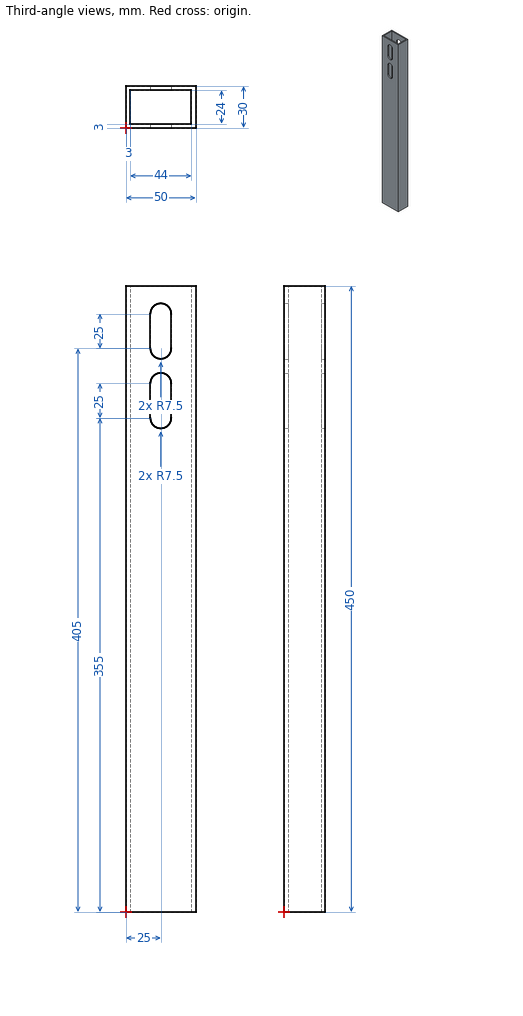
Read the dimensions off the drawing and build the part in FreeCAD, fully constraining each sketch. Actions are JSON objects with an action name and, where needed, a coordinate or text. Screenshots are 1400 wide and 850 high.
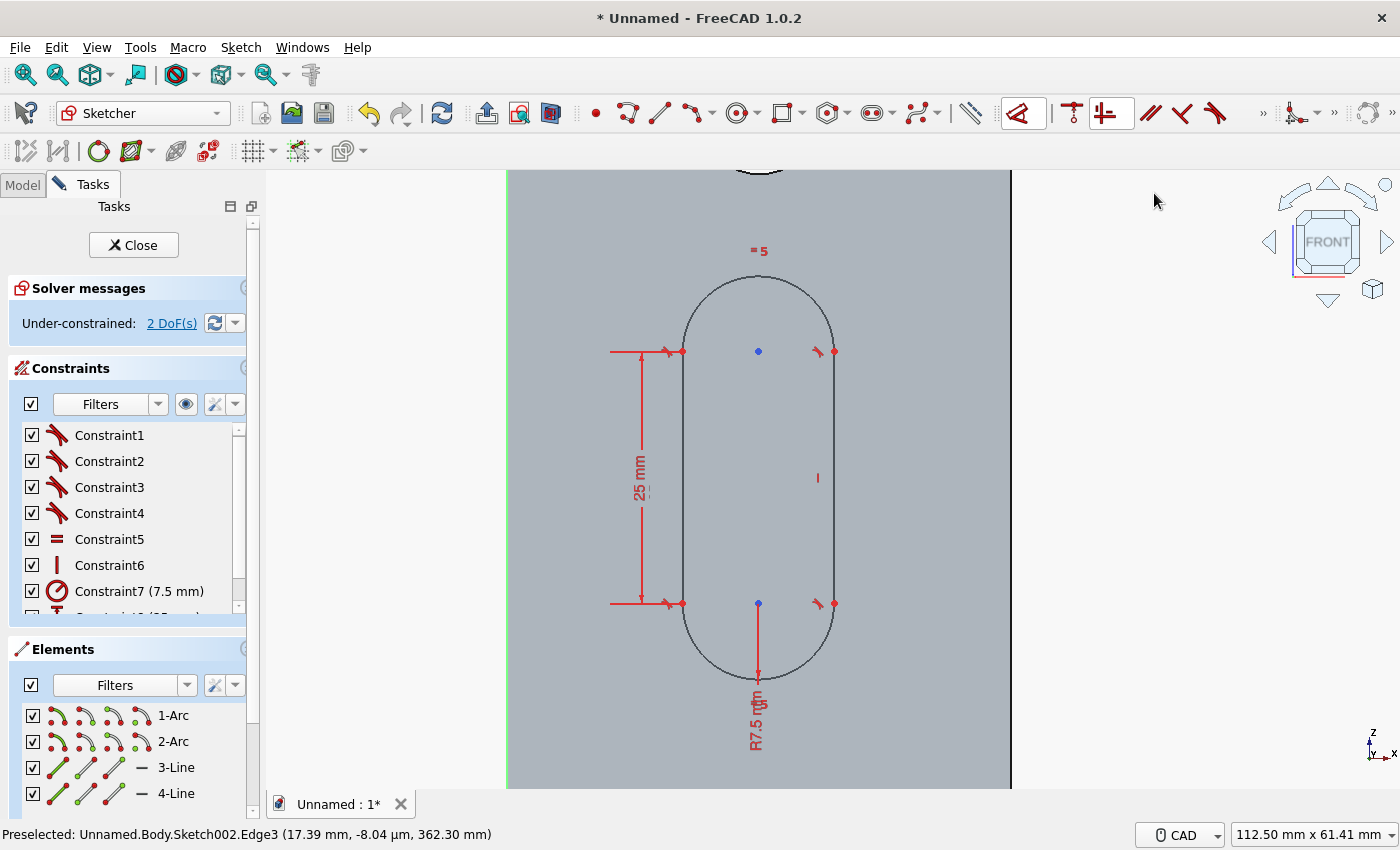
{"action": "left_click", "coordinate": [758, 604]}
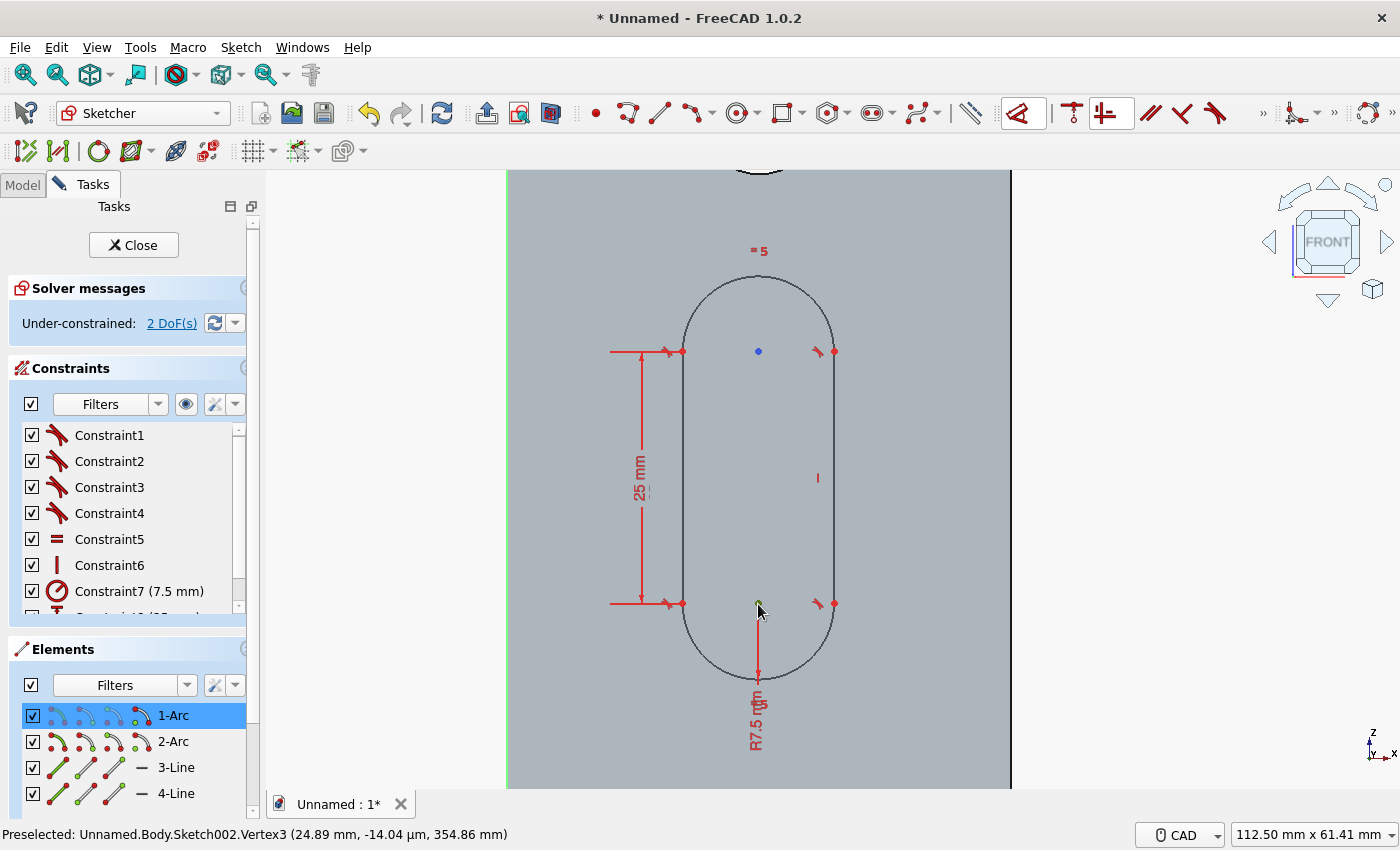
{"action": "left_click", "coordinate": [1040, 114]}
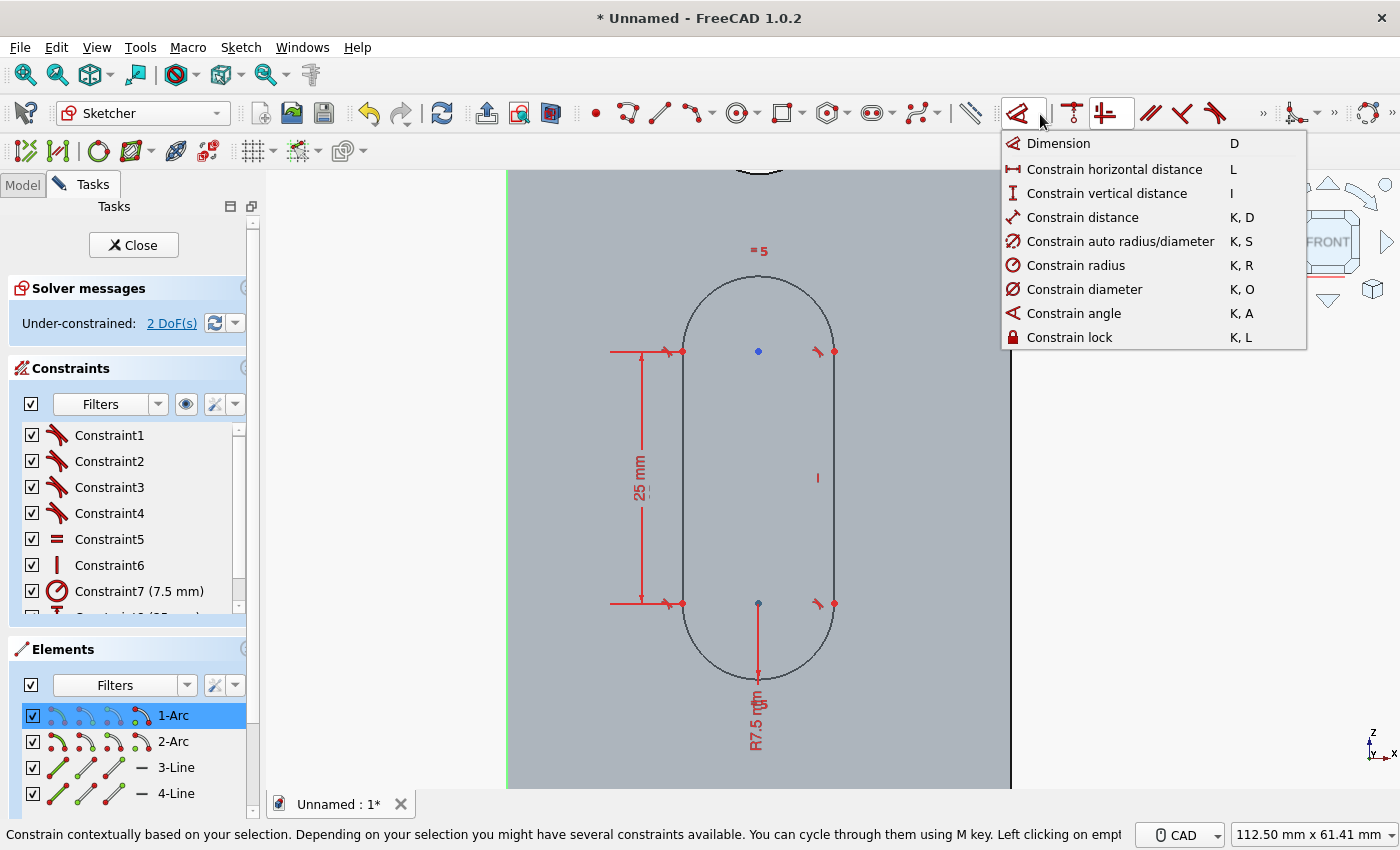
{"action": "left_click", "coordinate": [1154, 169]}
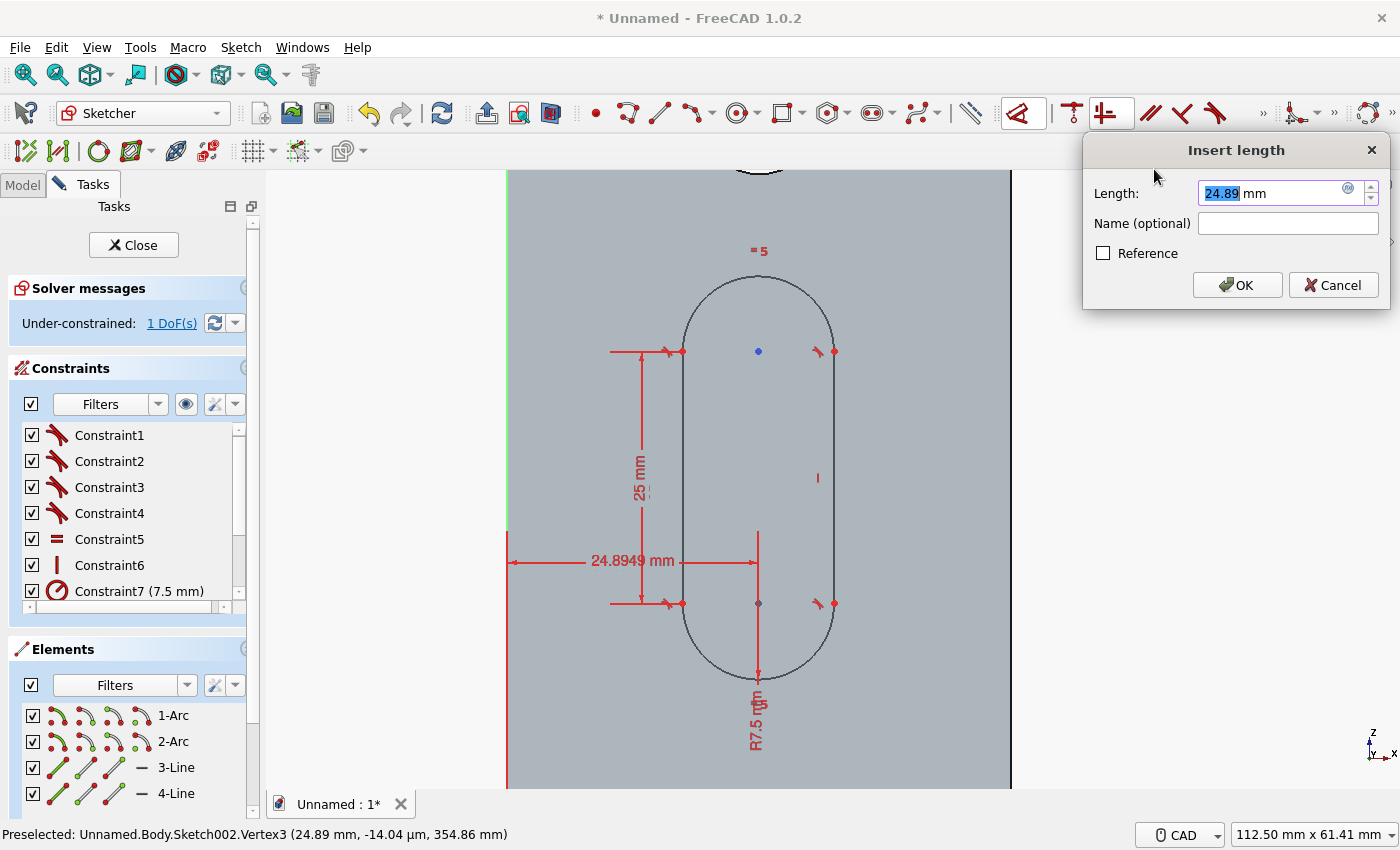
{"action": "type", "text": "25"}
{"action": "key", "text": "Return"}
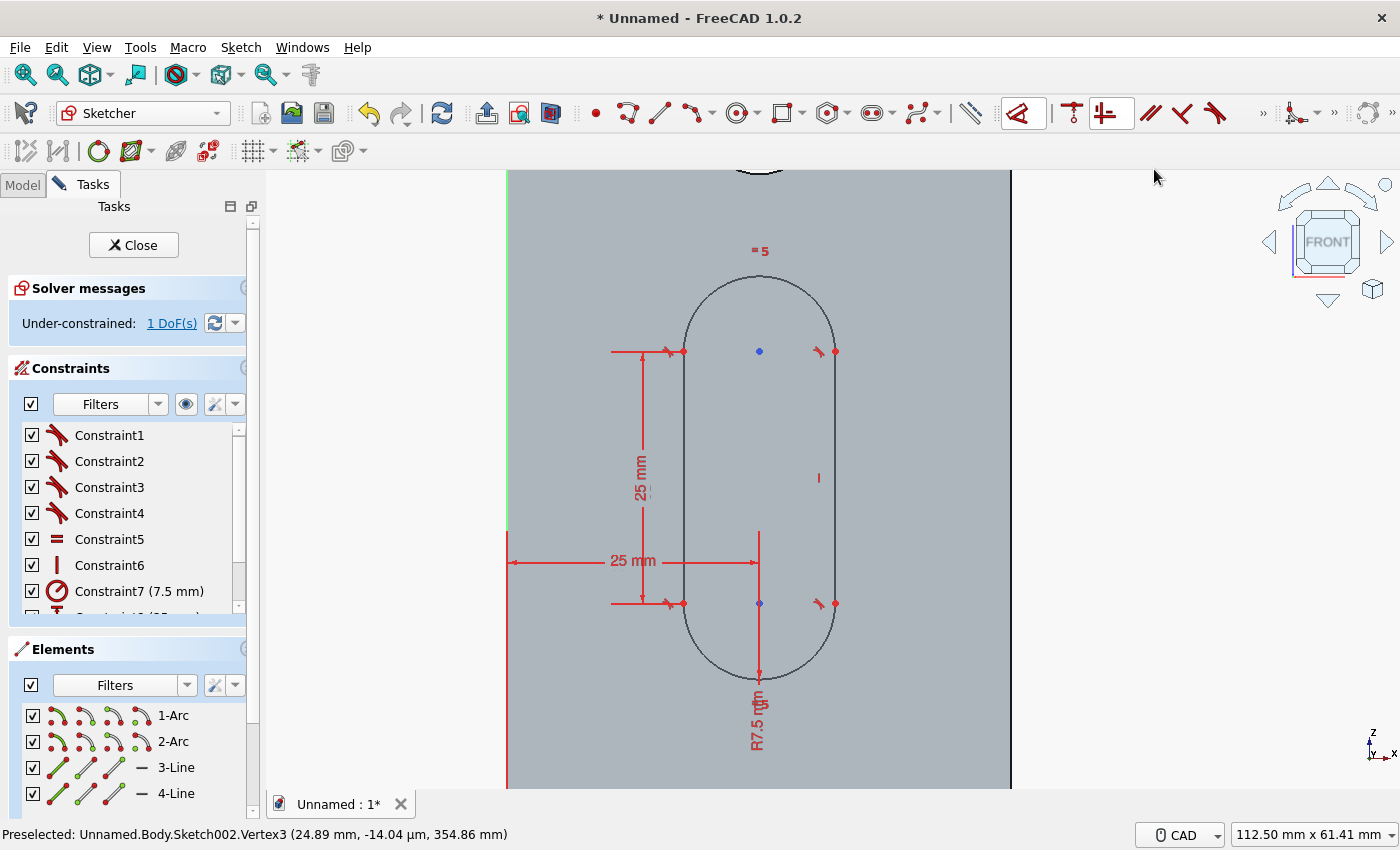
{"action": "left_click", "coordinate": [684, 604]}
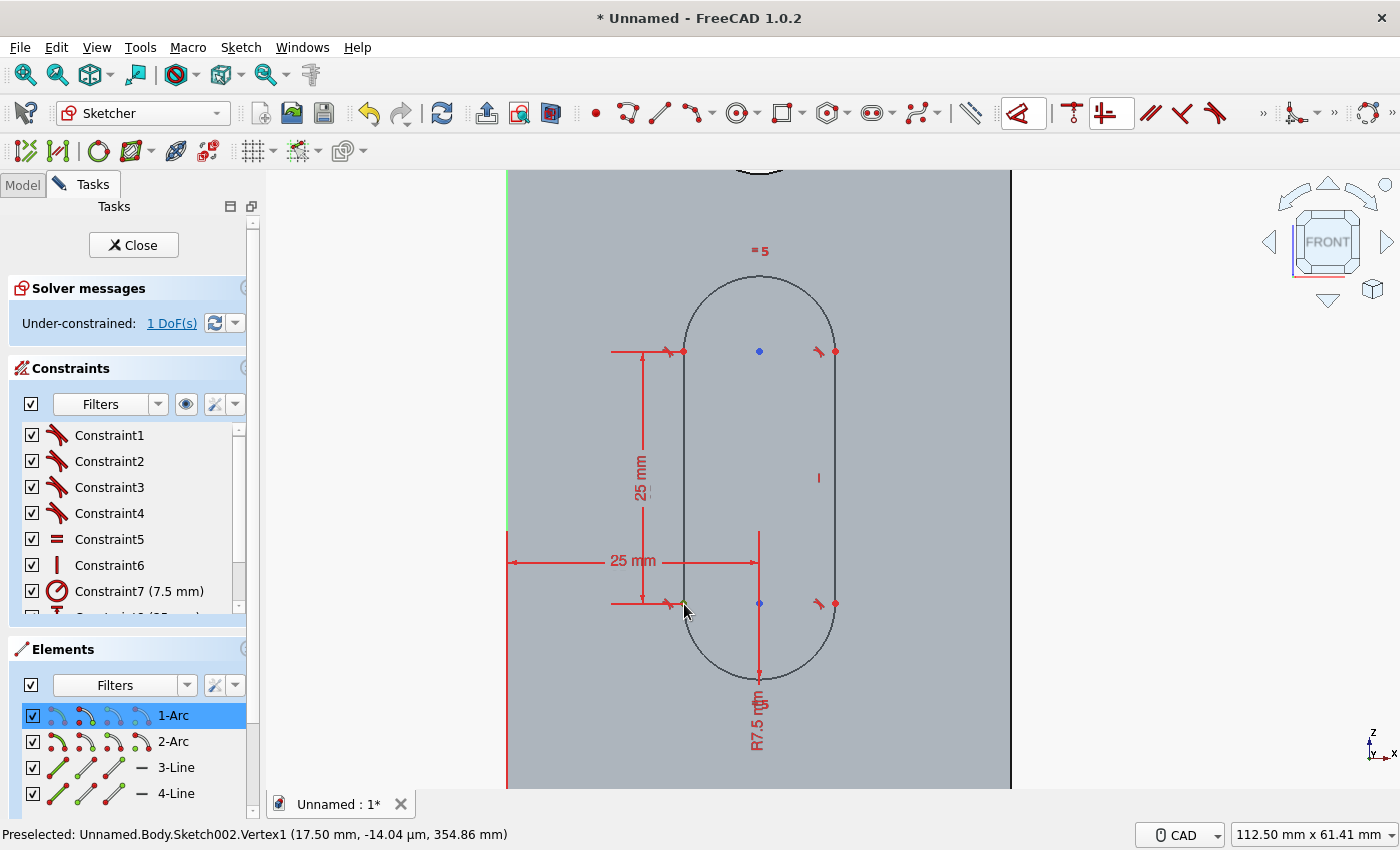
{"action": "key", "text": "i"}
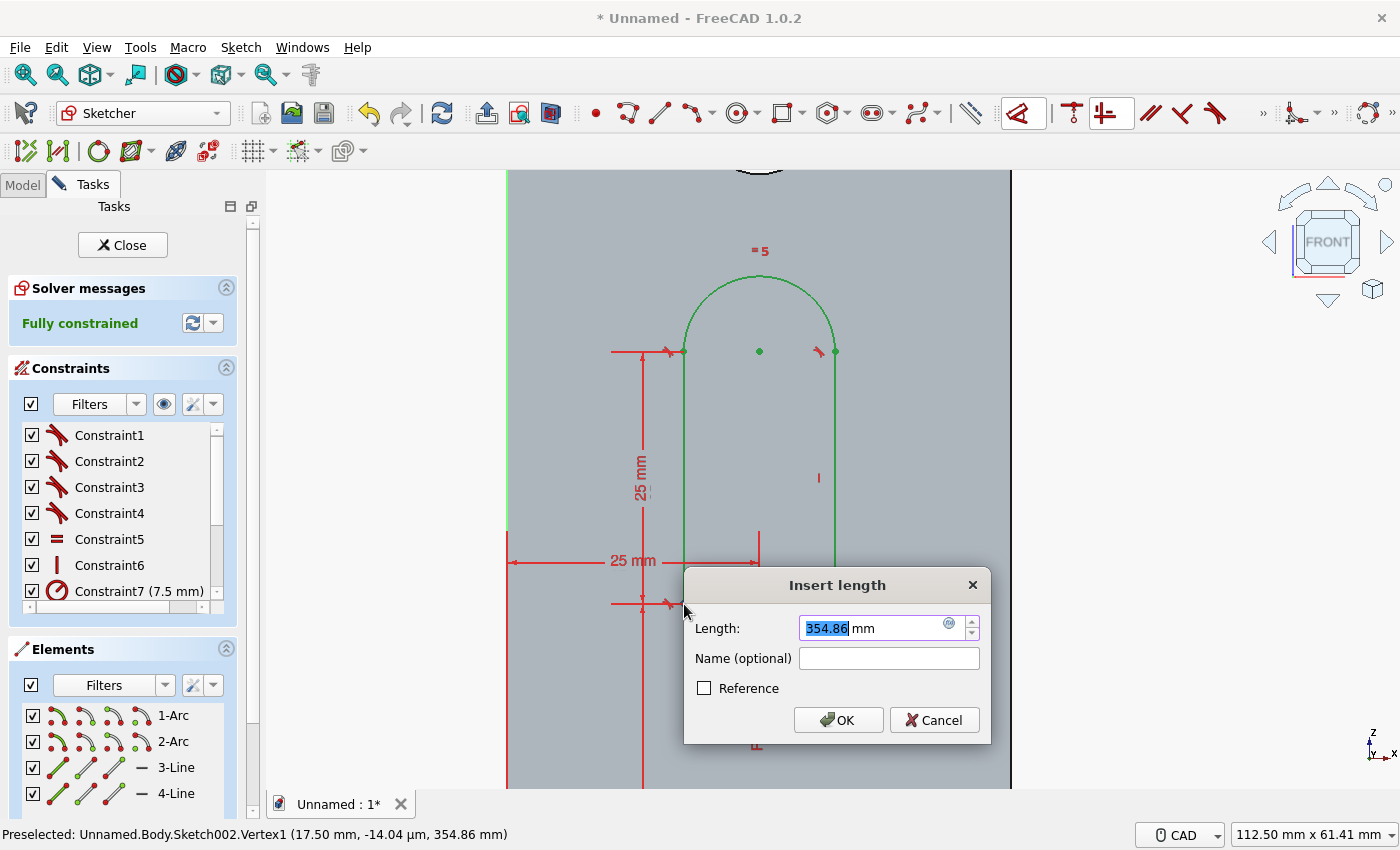
{"action": "type", "text": "355"}
{"action": "key", "text": "Return"}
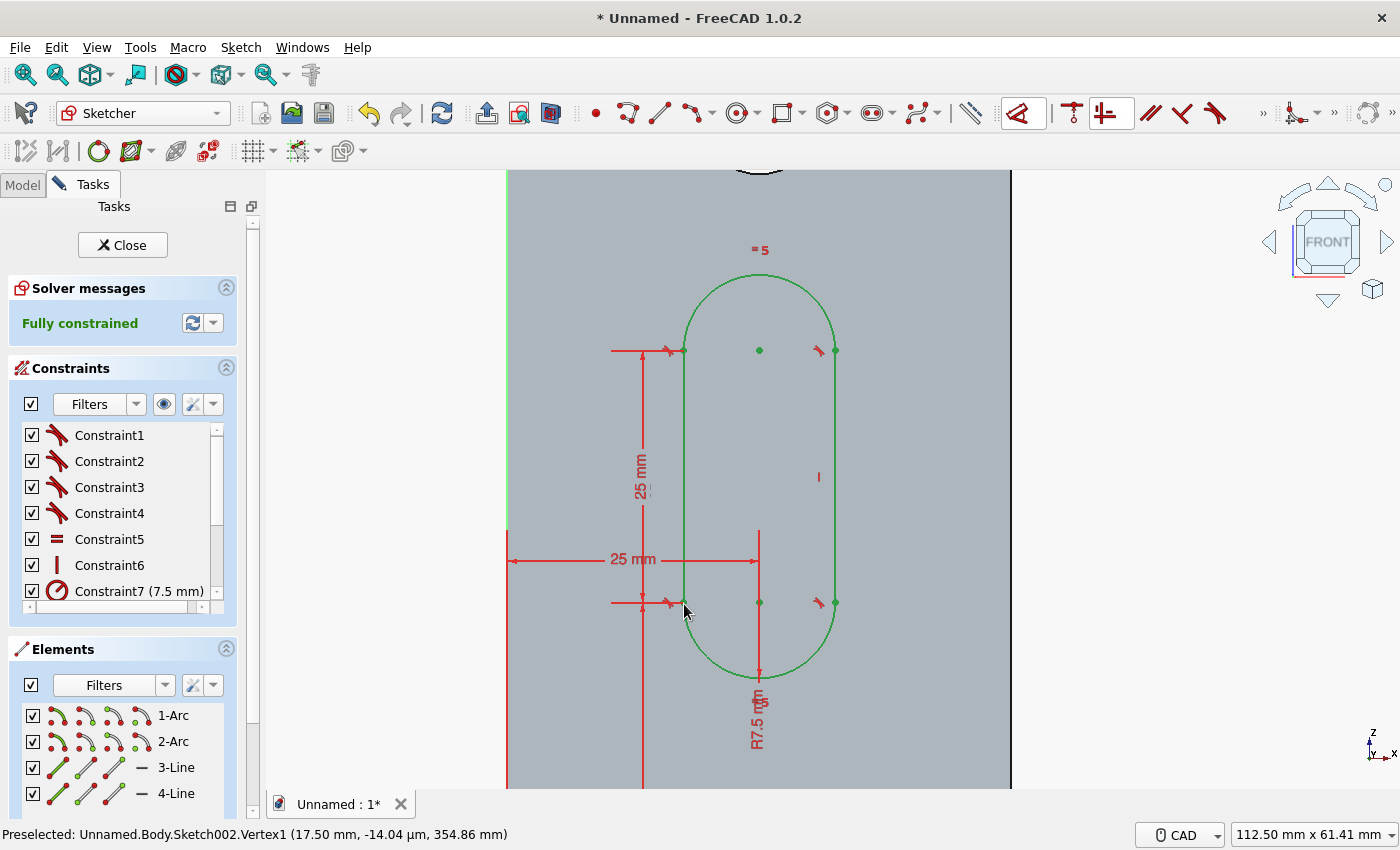
{"action": "left_click", "coordinate": [123, 245]}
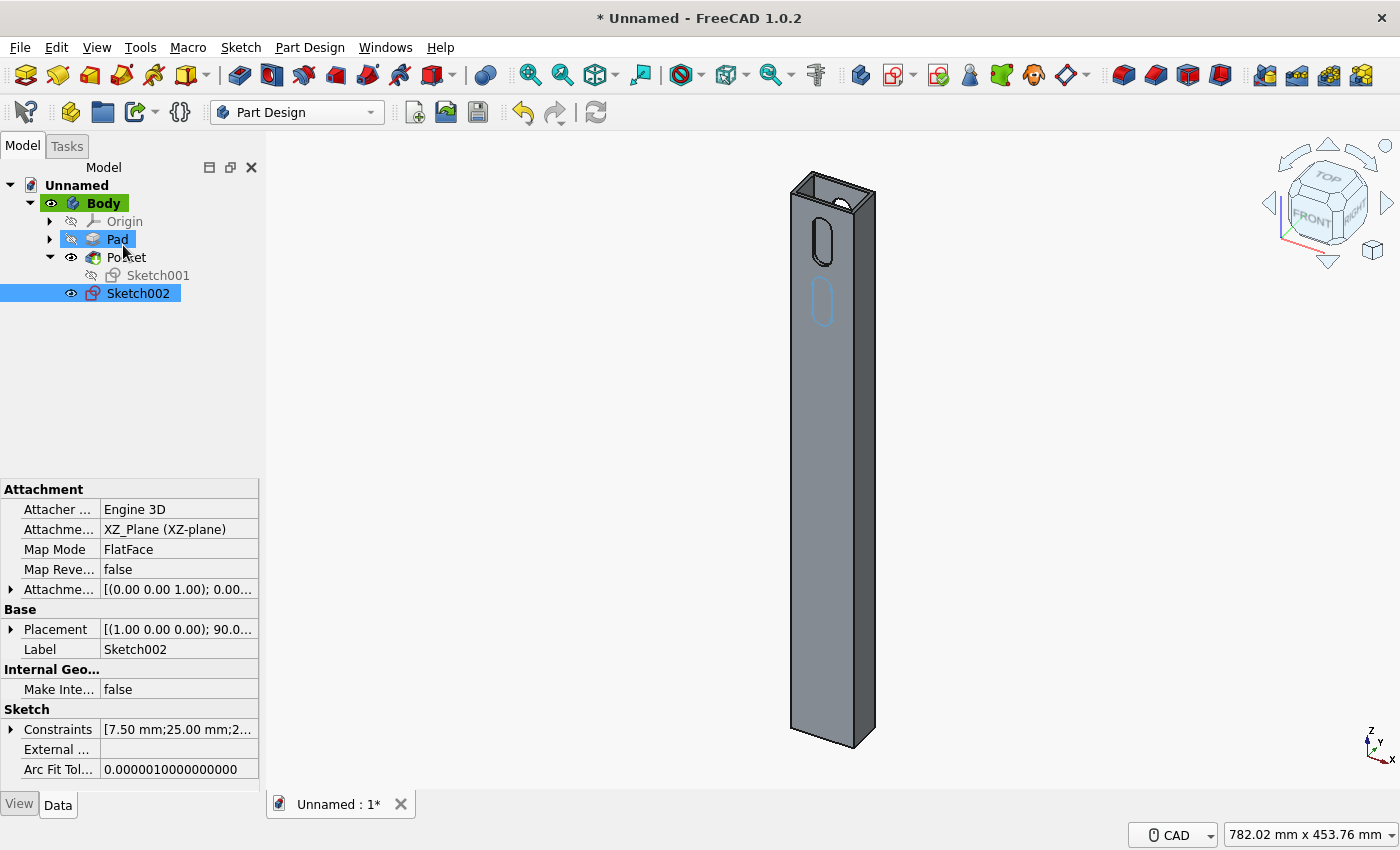
{"action": "left_click", "coordinate": [240, 76]}